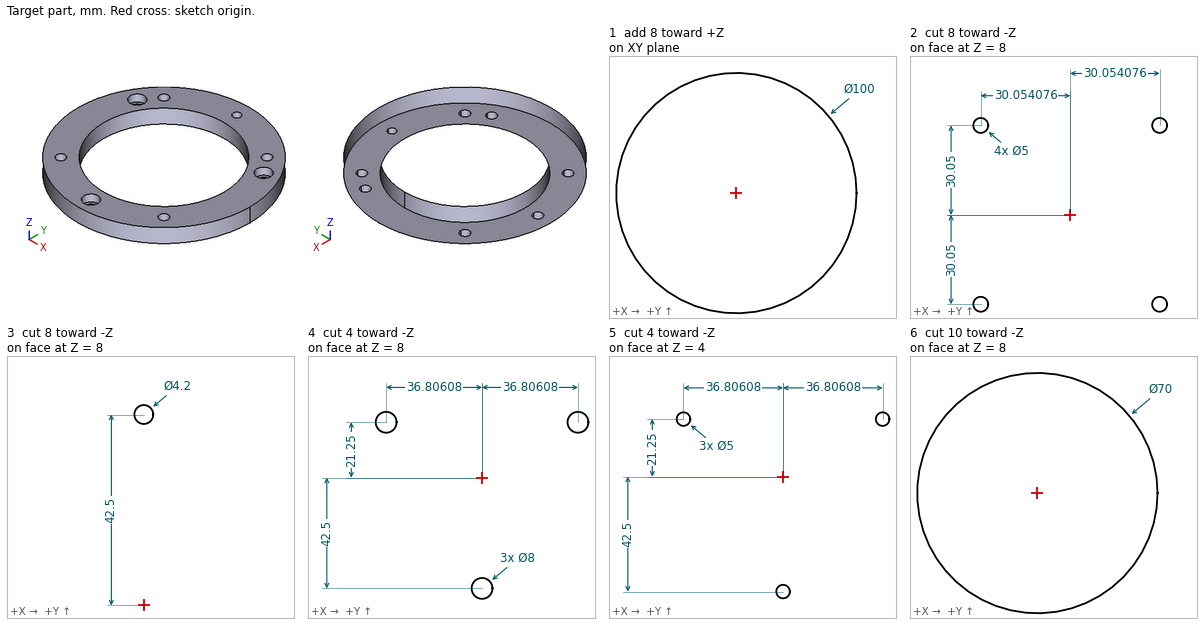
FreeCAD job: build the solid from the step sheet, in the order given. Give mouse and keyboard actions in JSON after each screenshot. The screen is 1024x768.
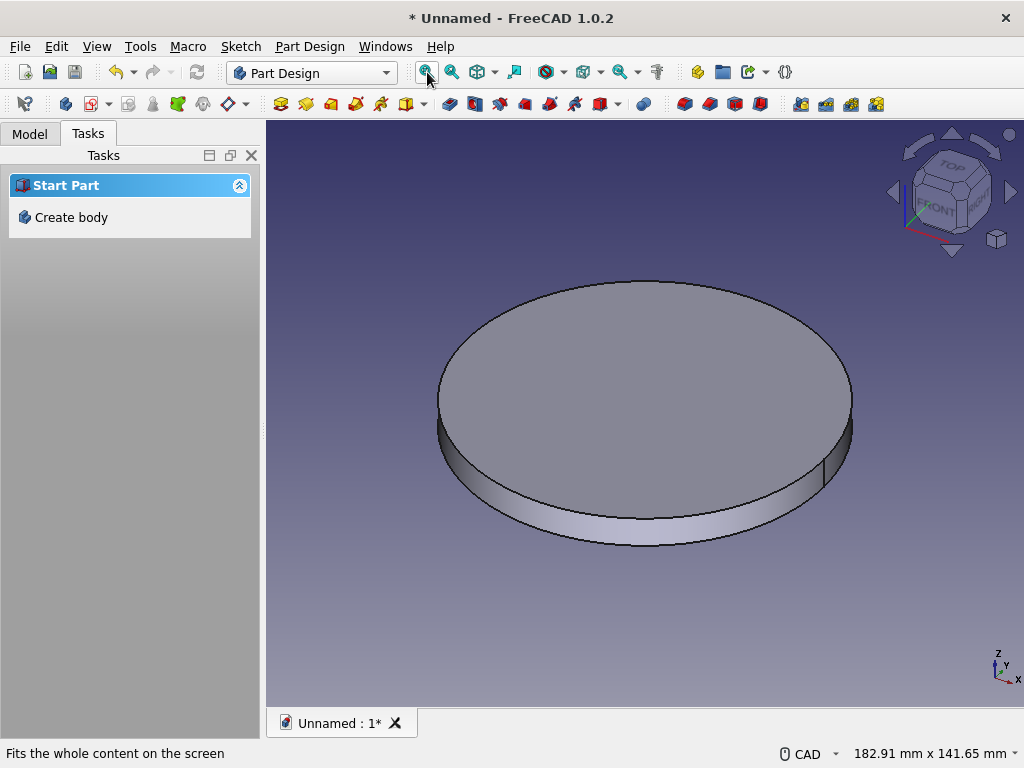
{"action": "left_click", "coordinate": [645, 399]}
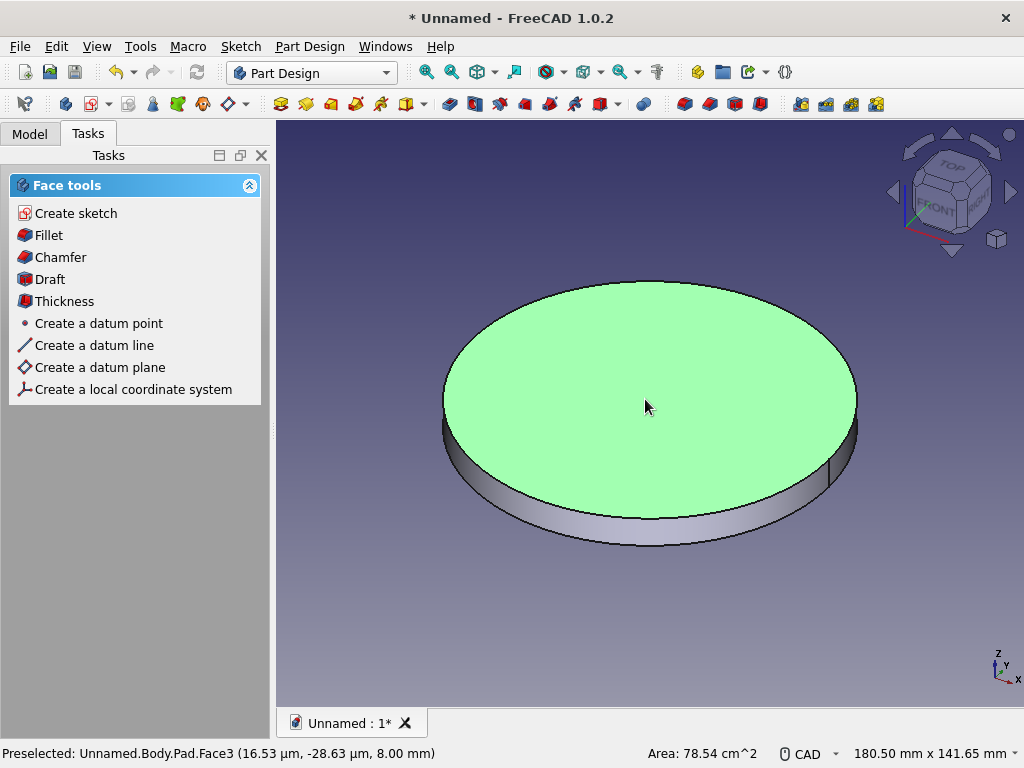
{"action": "left_click", "coordinate": [90, 104]}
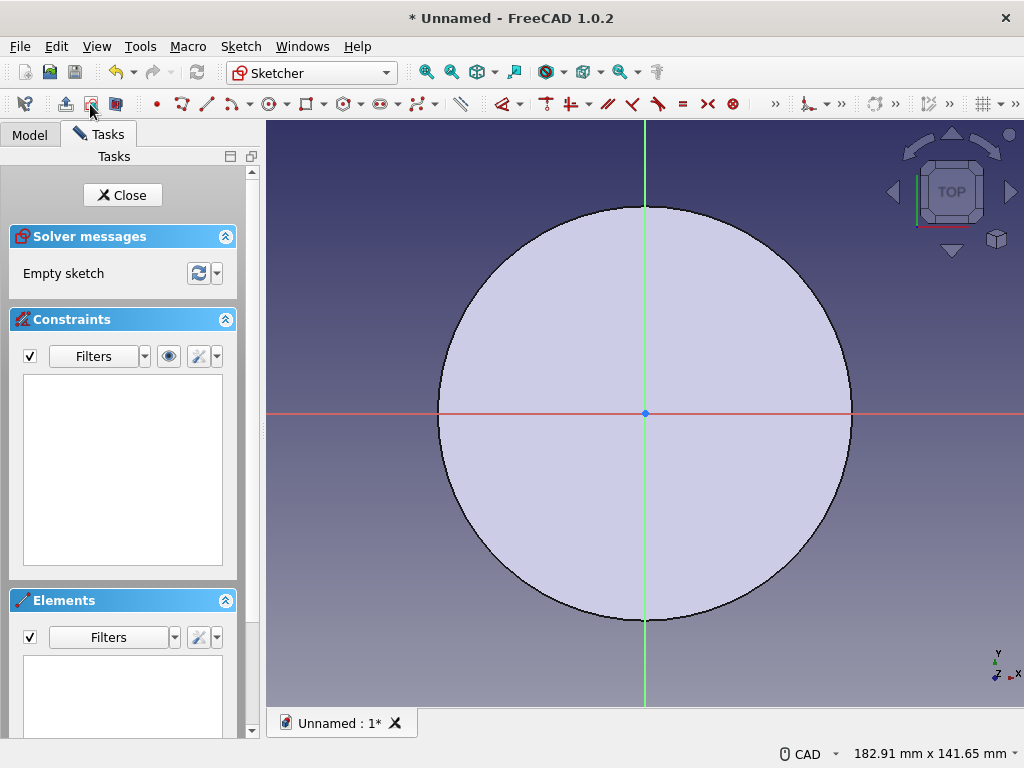
{"action": "scroll", "coordinate": [784, 413], "scroll_direction": "up", "scroll_amount": 2}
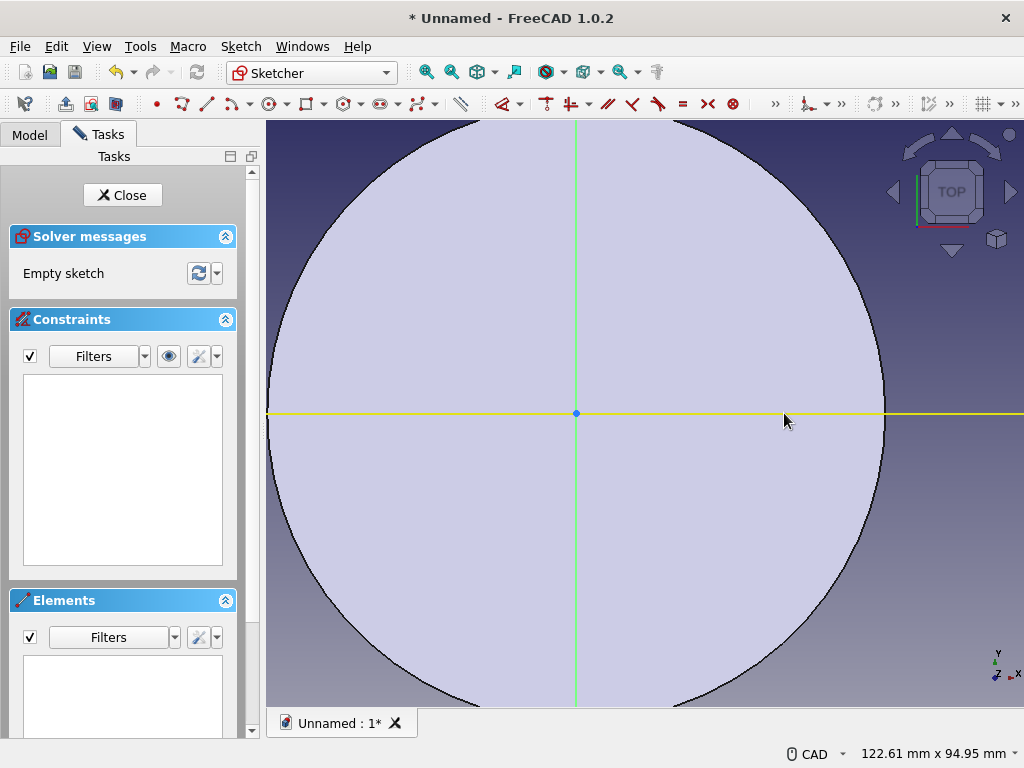
{"action": "left_click", "coordinate": [268, 104]}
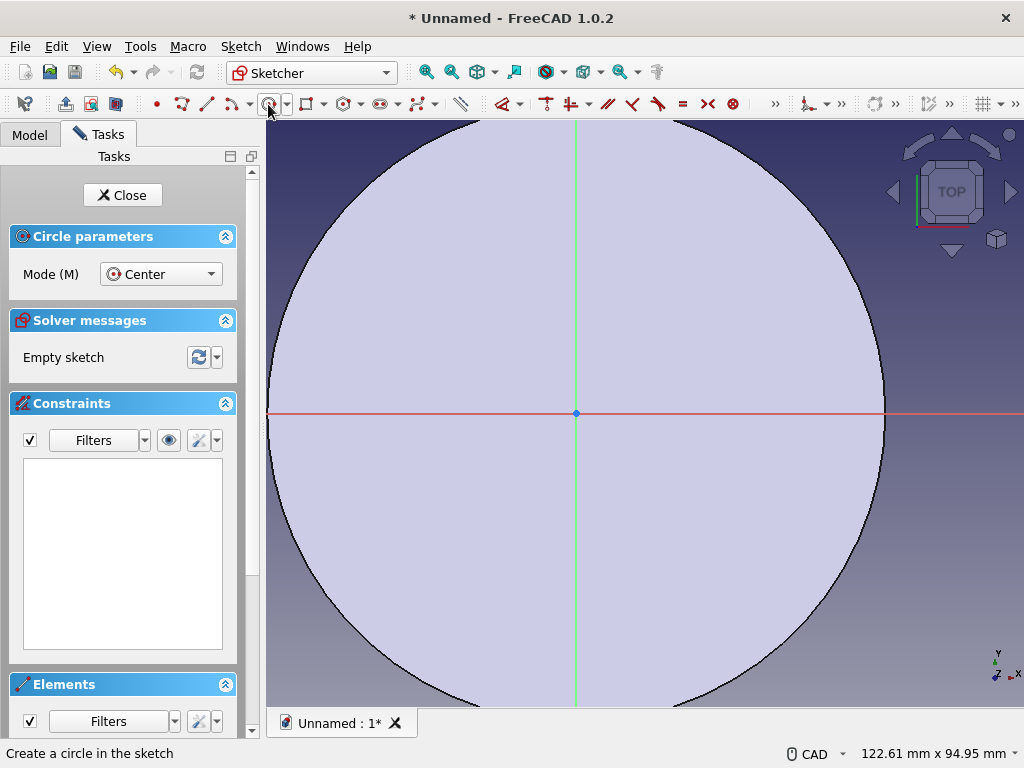
{"action": "scroll", "coordinate": [390, 228], "scroll_direction": "up", "scroll_amount": 2}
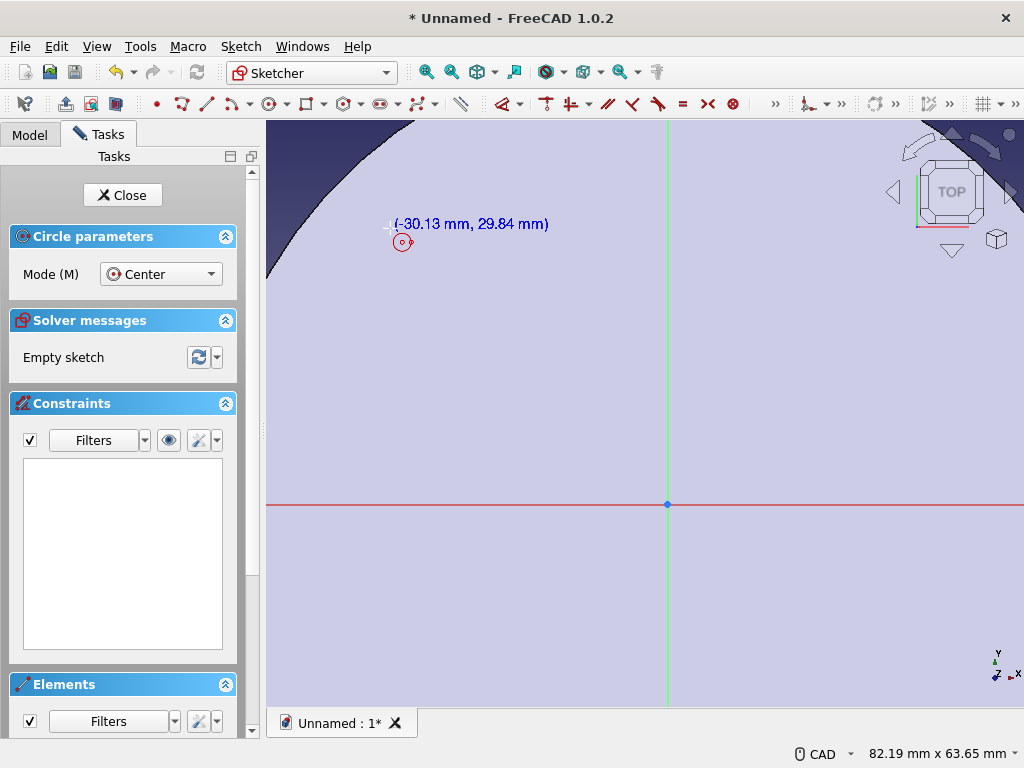
{"action": "left_click", "coordinate": [391, 227]}
{"action": "mouse_move", "coordinate": [407, 211]}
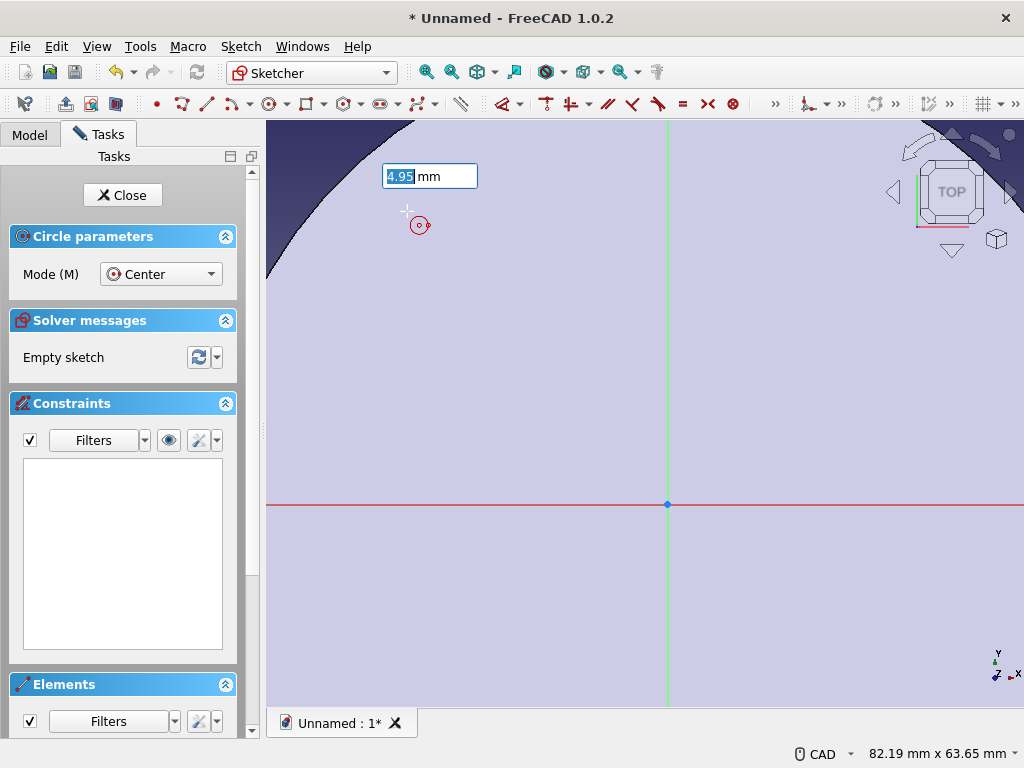
{"action": "type", "text": "5"}
{"action": "key", "text": "Return"}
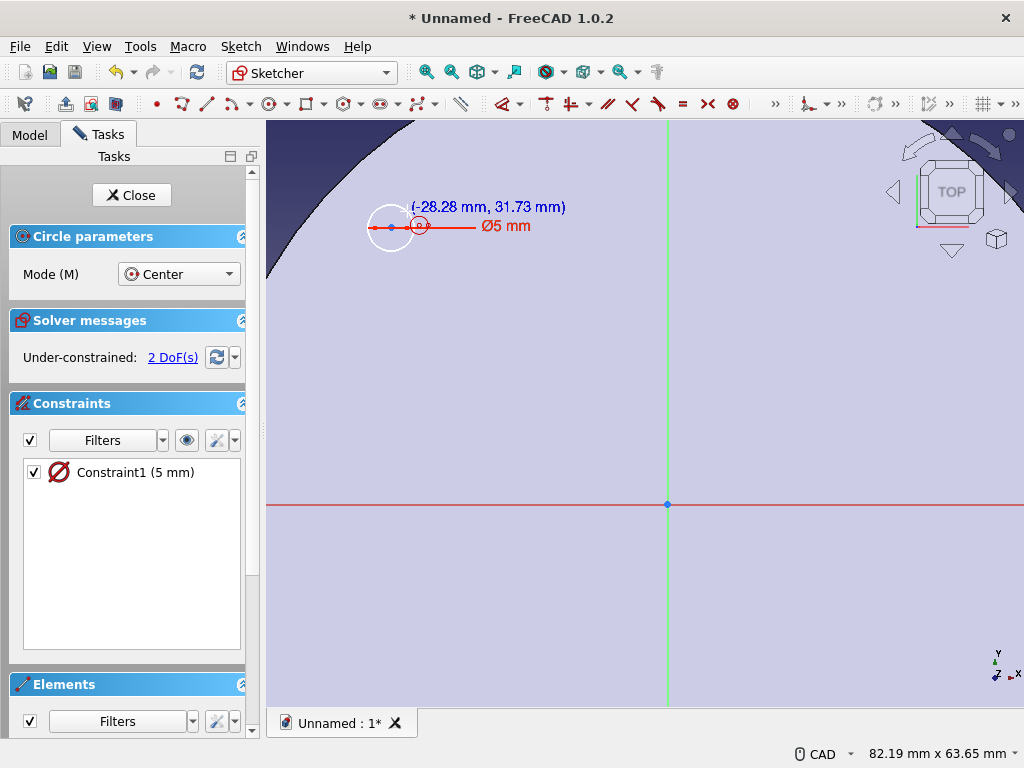
{"action": "scroll", "coordinate": [391, 228], "scroll_direction": "down", "scroll_amount": 2}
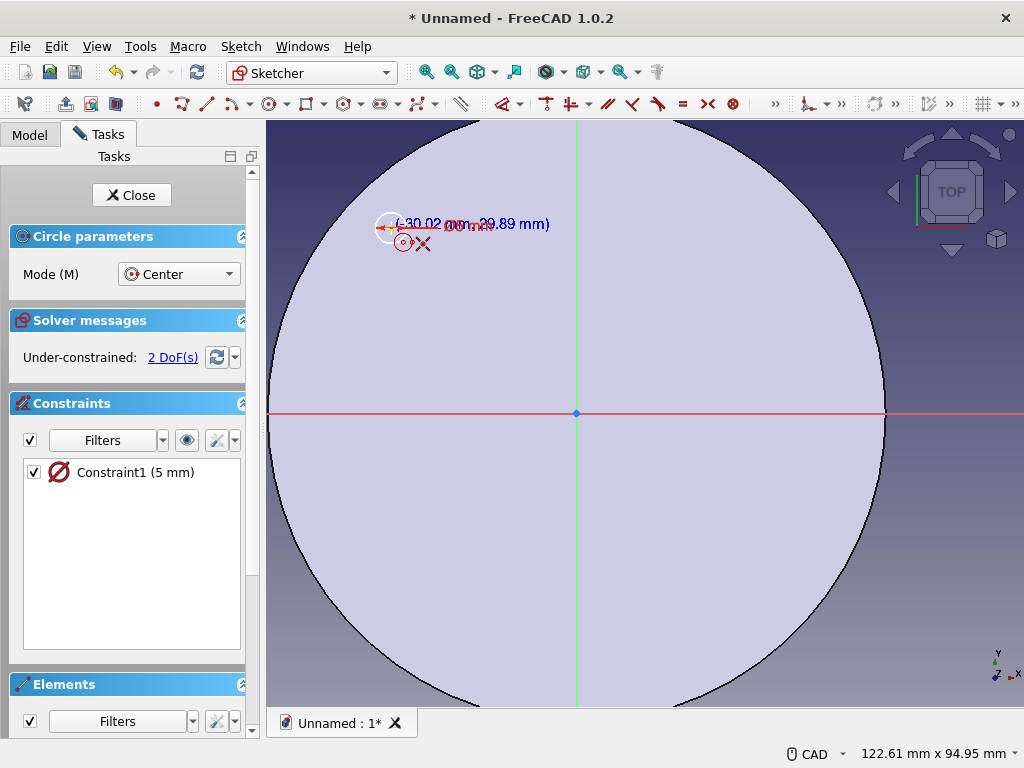
{"action": "scroll", "coordinate": [762, 228], "scroll_direction": "up", "scroll_amount": 2}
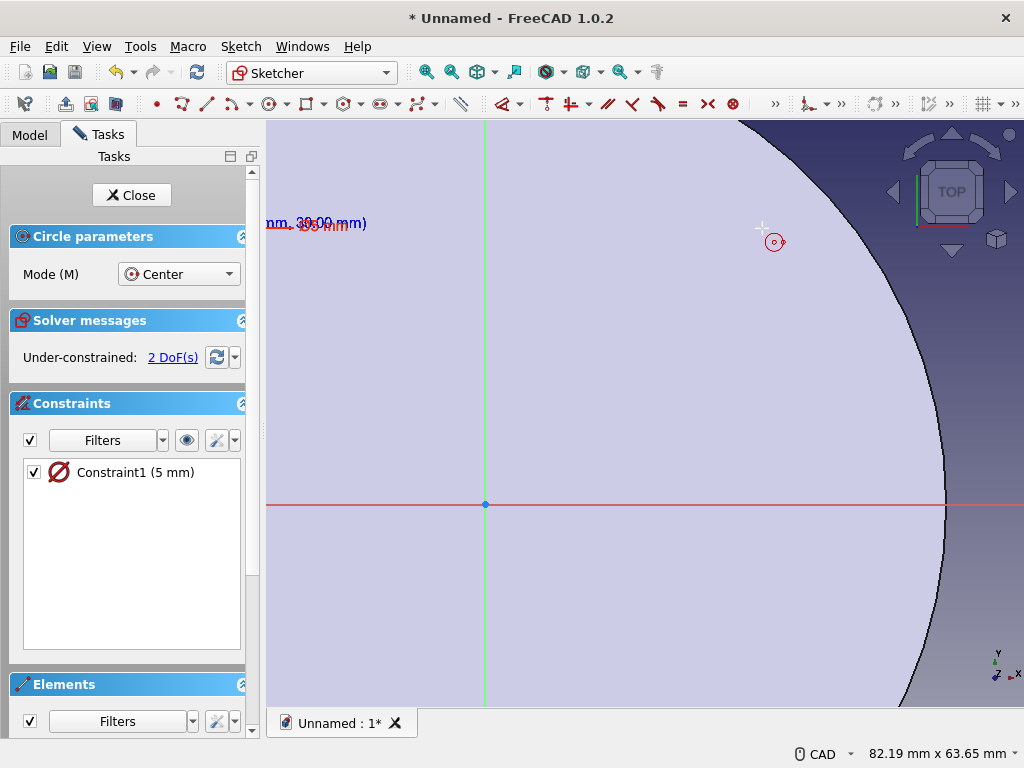
{"action": "left_click", "coordinate": [762, 227]}
{"action": "mouse_move", "coordinate": [779, 211]}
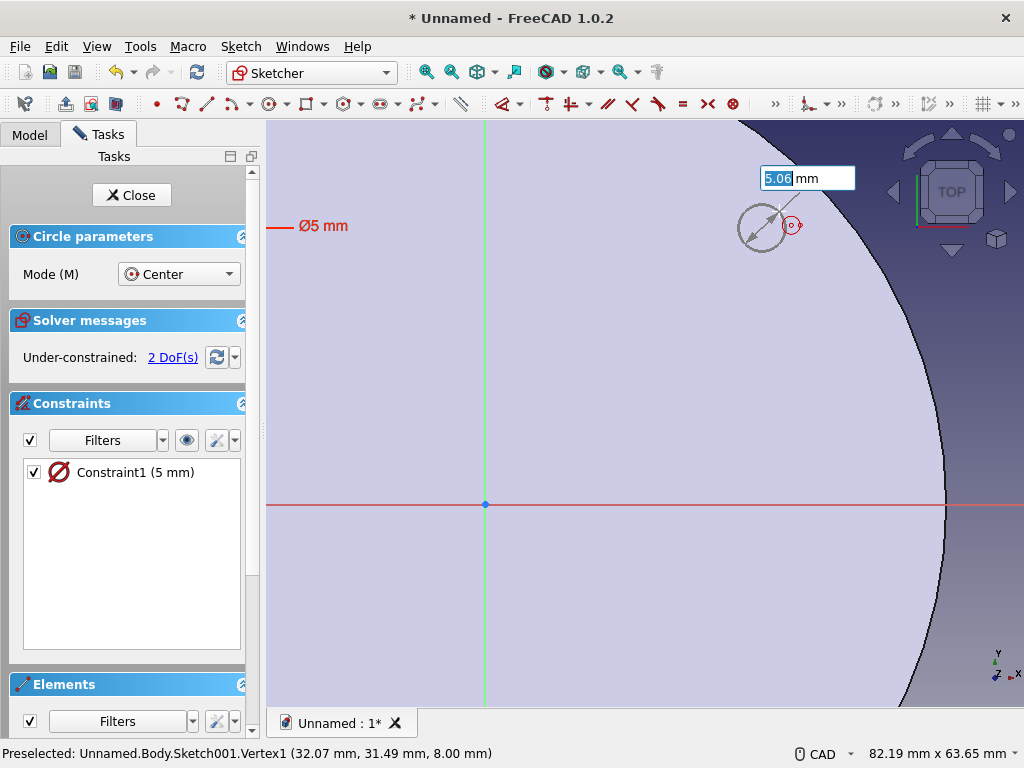
{"action": "type", "text": "5"}
{"action": "key", "text": "Return"}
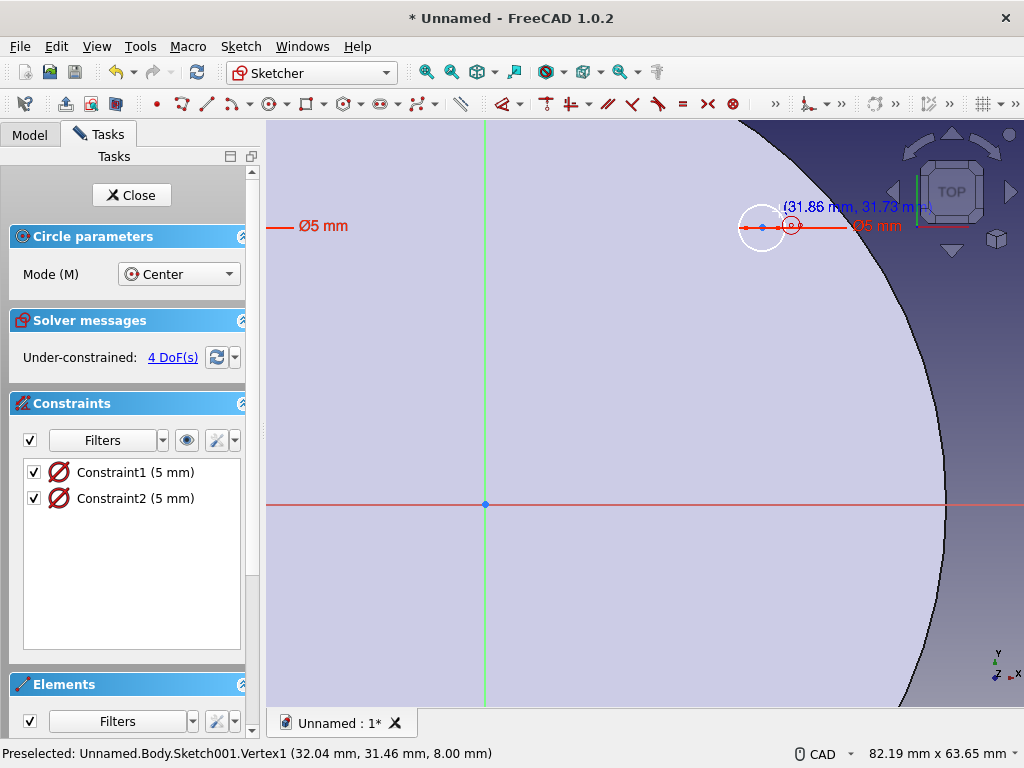
{"action": "scroll", "coordinate": [762, 228], "scroll_direction": "down", "scroll_amount": 2}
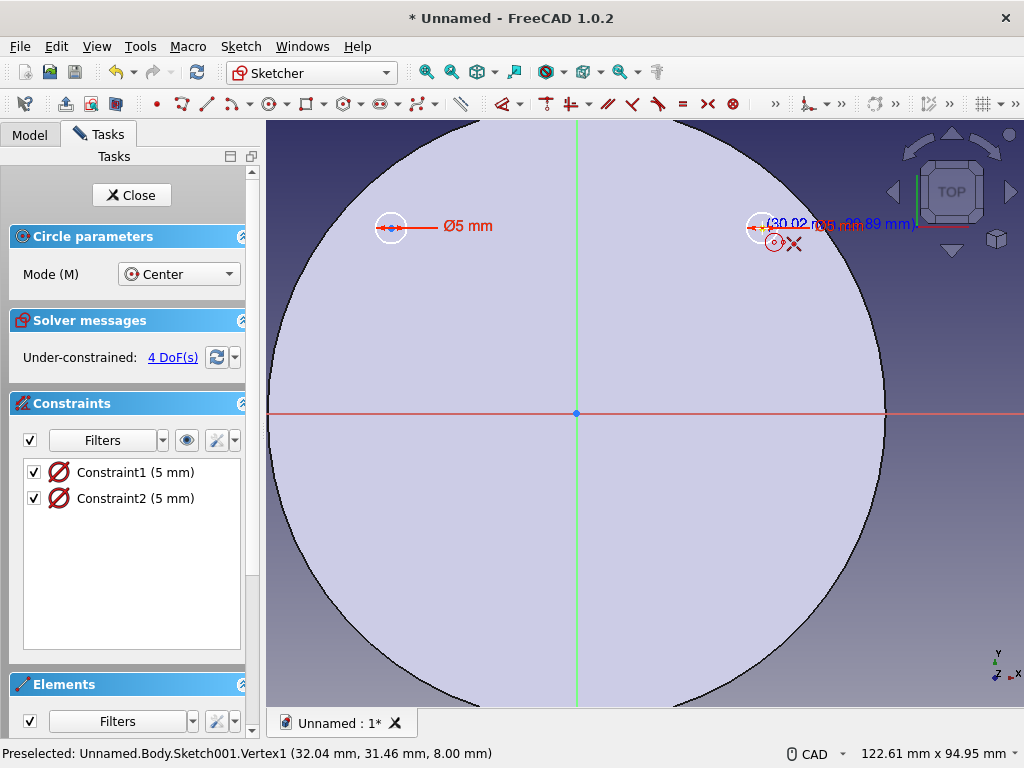
{"action": "scroll", "coordinate": [391, 599], "scroll_direction": "up", "scroll_amount": 2}